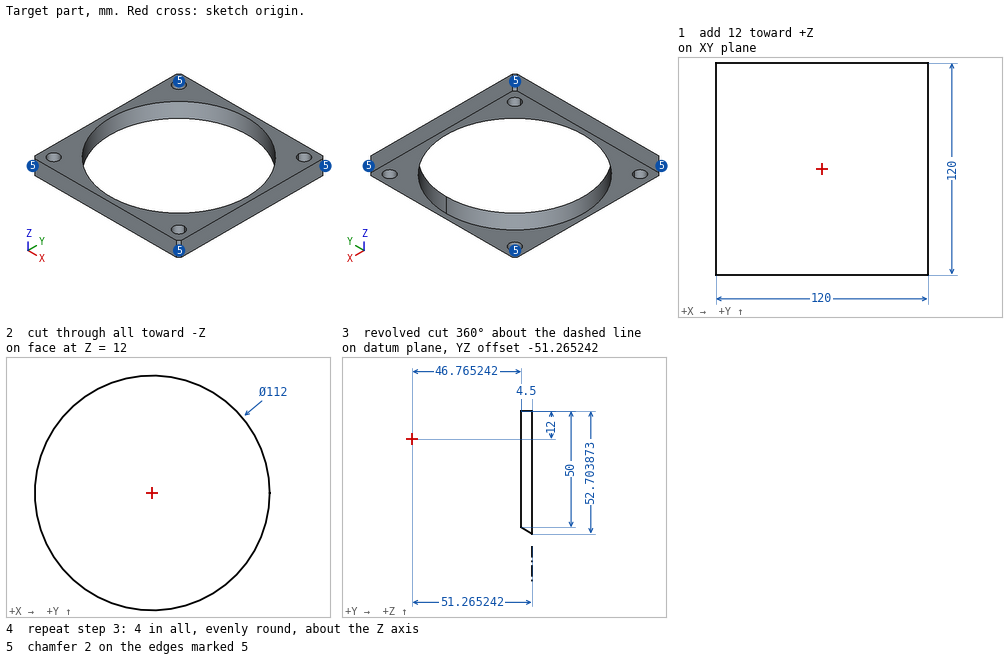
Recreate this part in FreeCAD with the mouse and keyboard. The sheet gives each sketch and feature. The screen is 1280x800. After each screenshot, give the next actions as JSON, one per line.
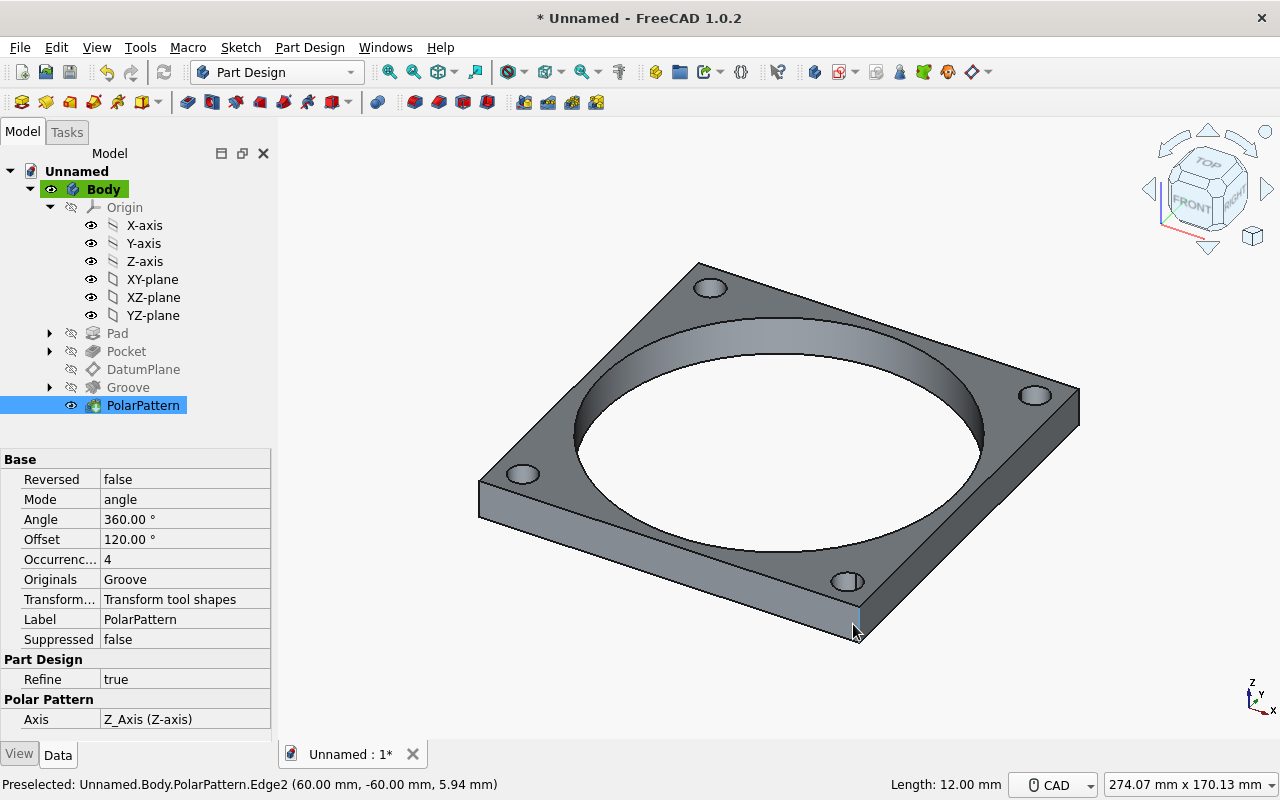
{"action": "key", "text": "0"}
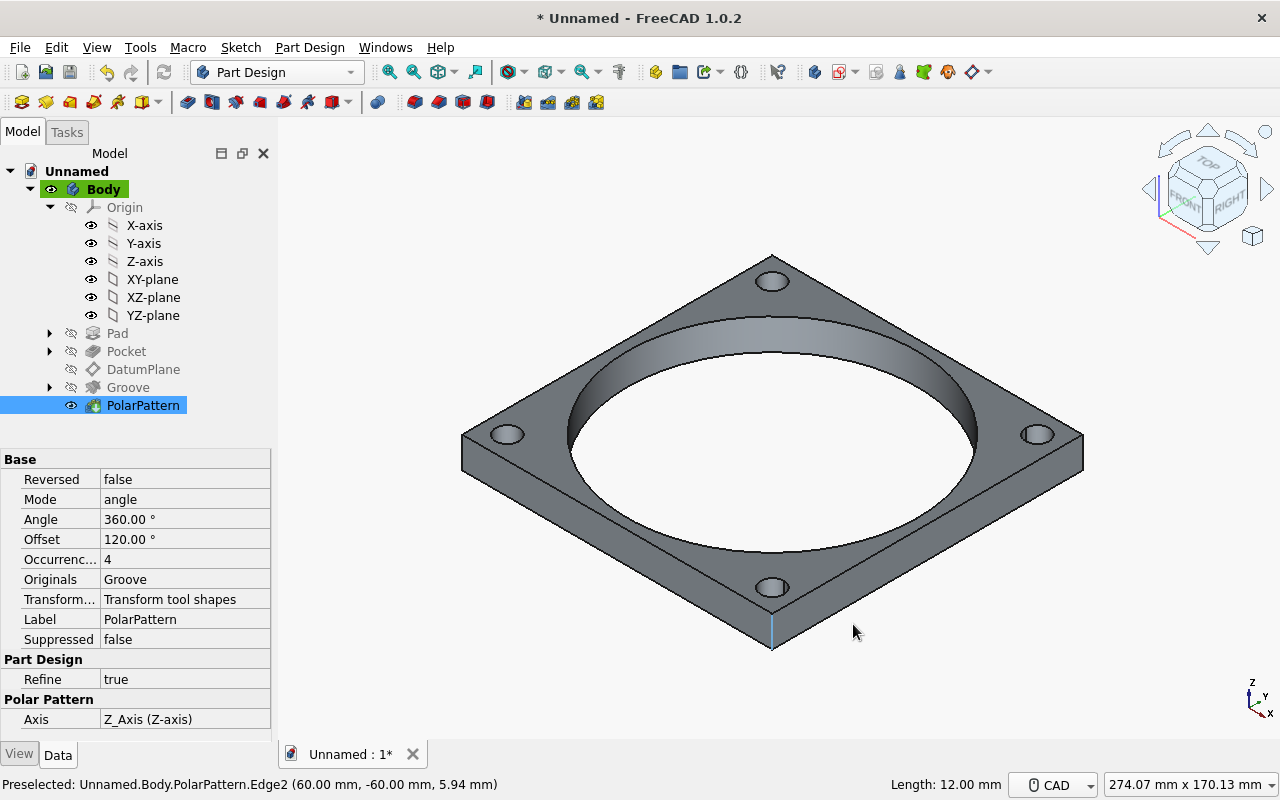
{"action": "key", "text": "2"}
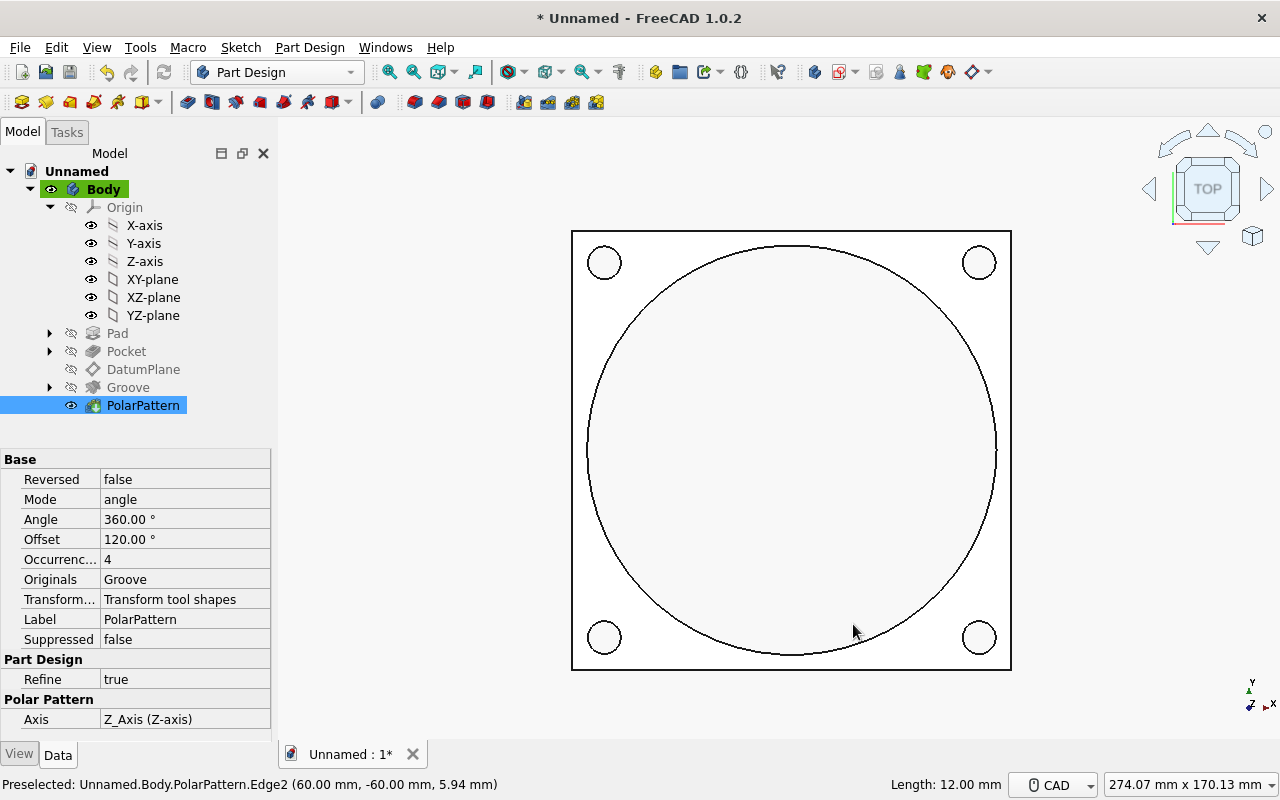
{"action": "key", "text": "1"}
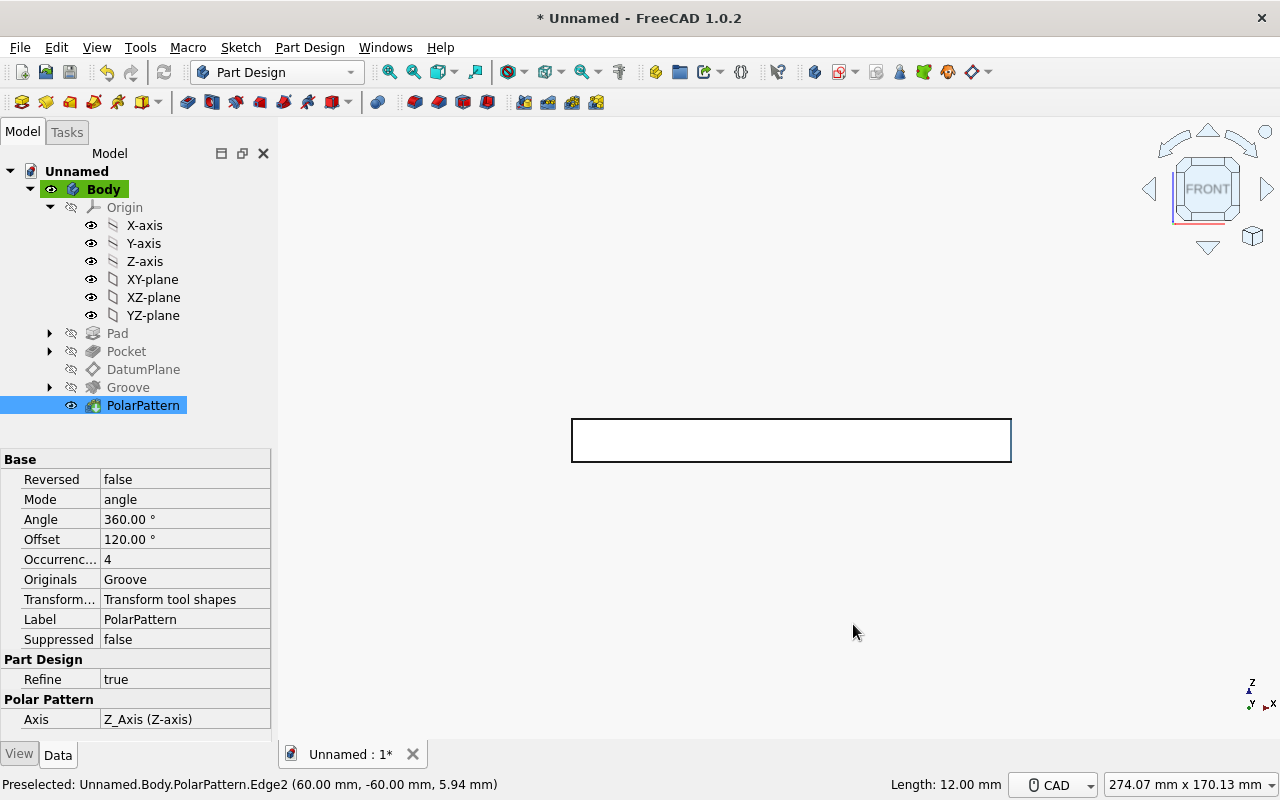
{"action": "left_click", "coordinate": [390, 72]}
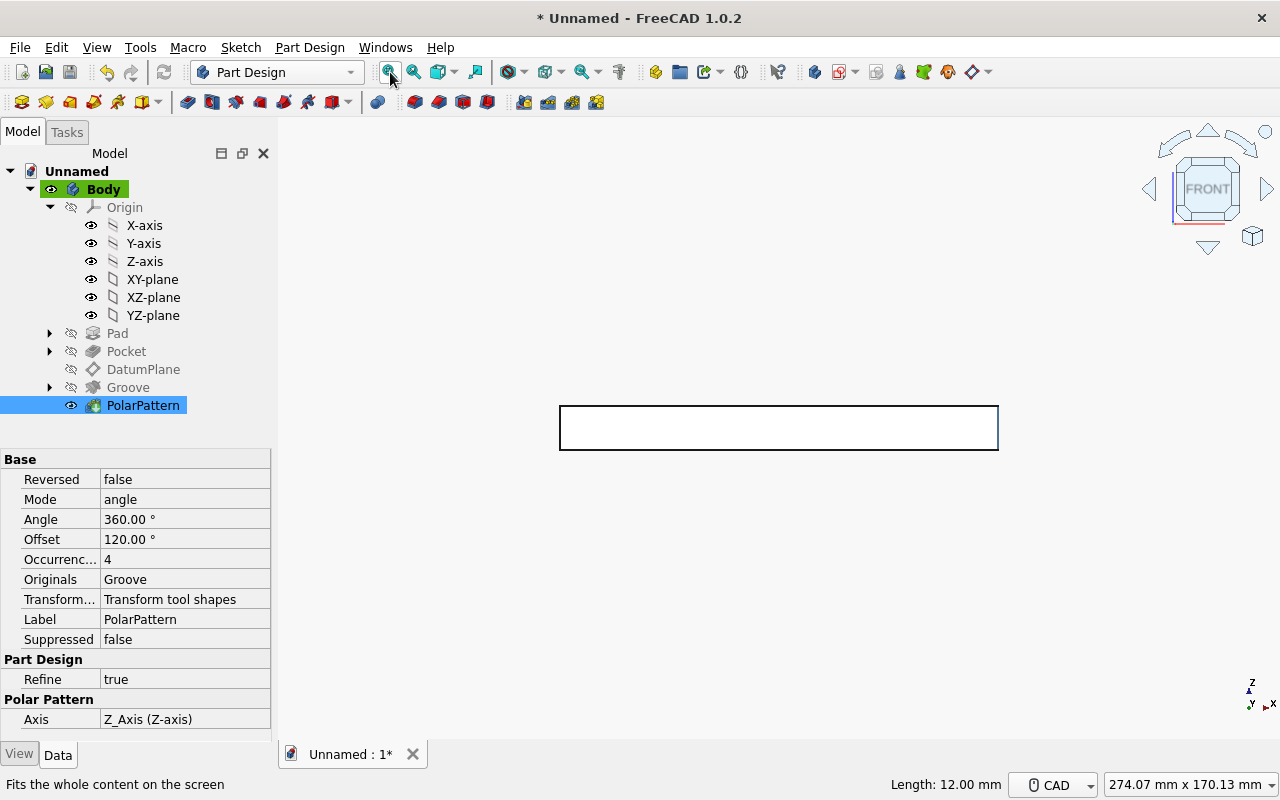
{"action": "left_click", "coordinate": [560, 427], "text": "ctrl"}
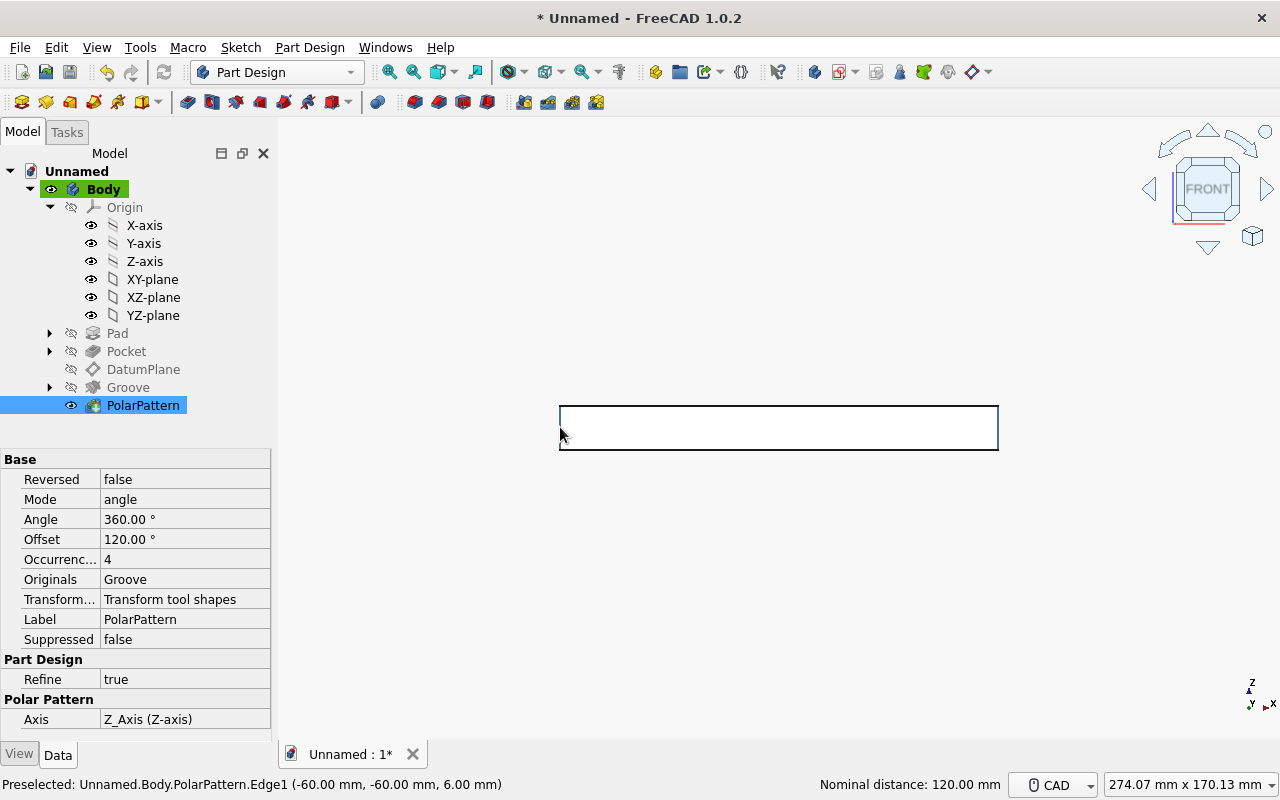
{"action": "key", "text": "3"}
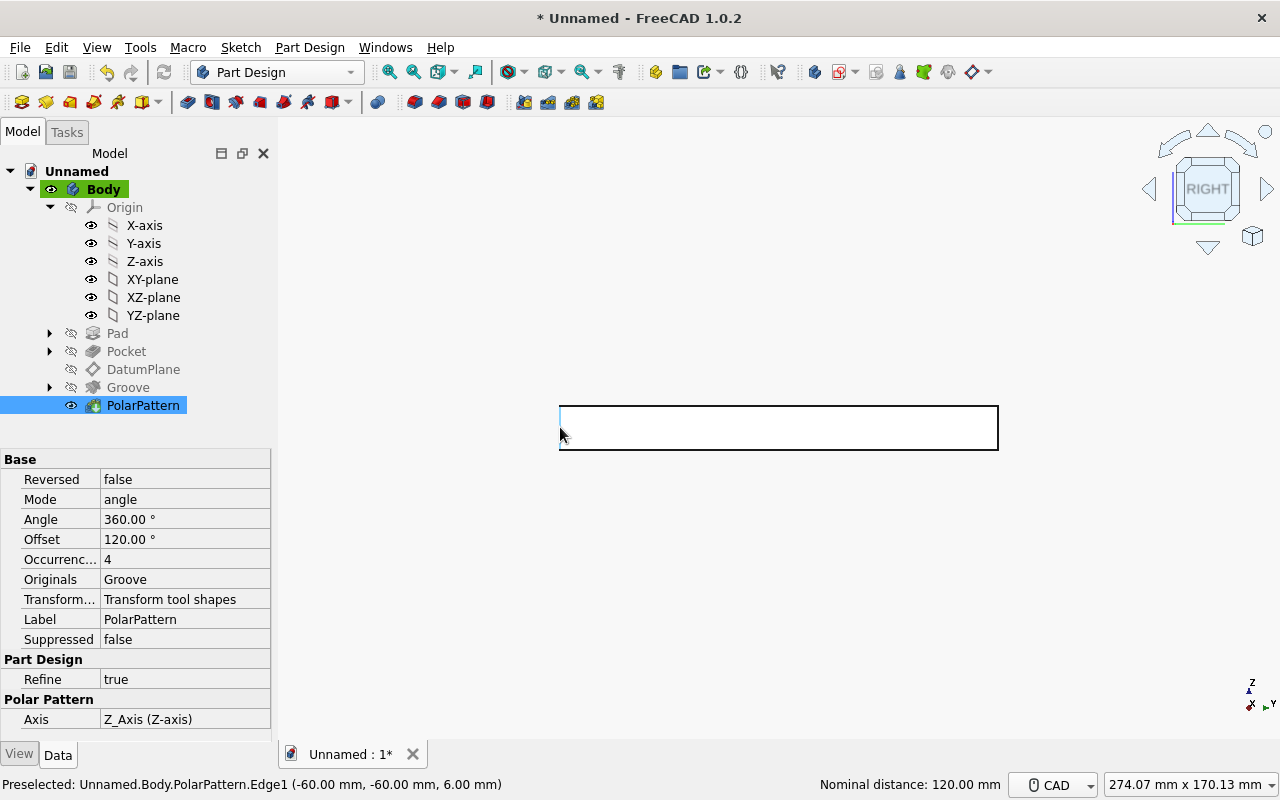
{"action": "key", "text": "v f"}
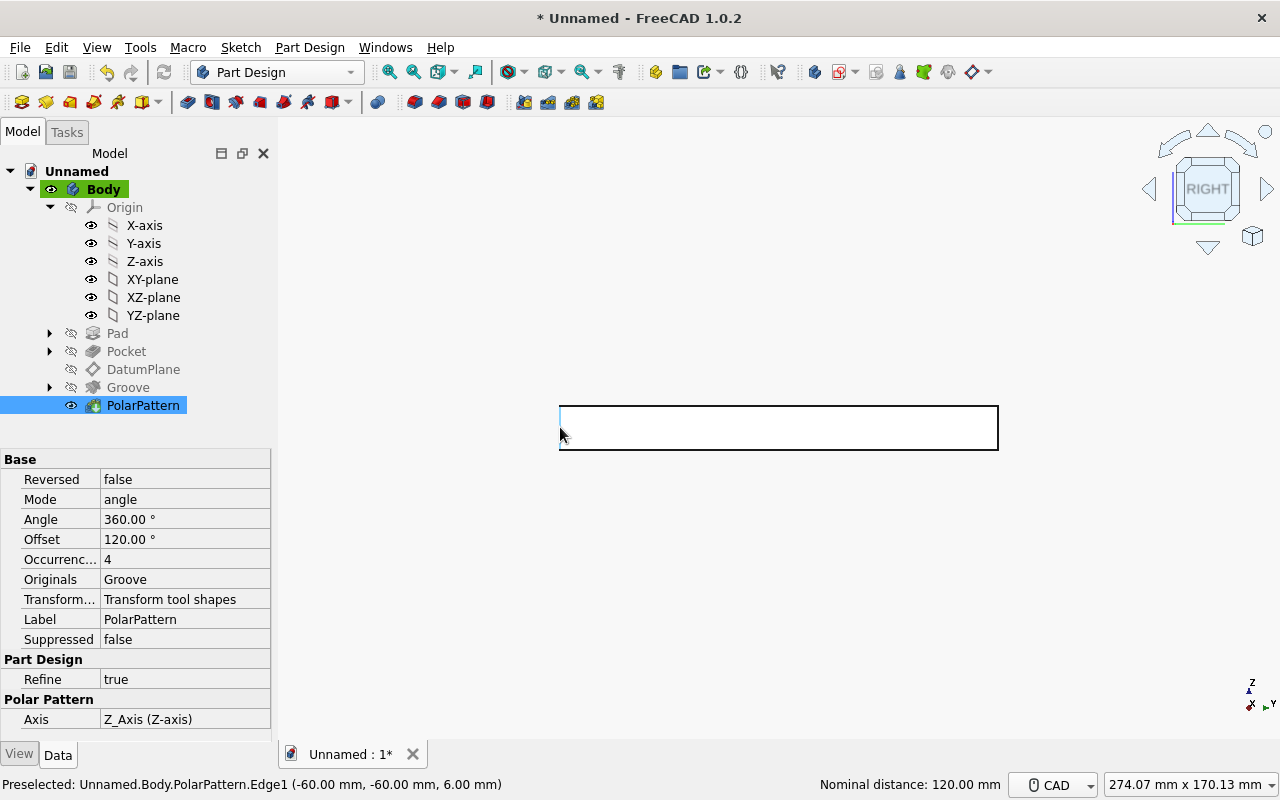
{"action": "left_click", "coordinate": [998, 427], "text": "ctrl"}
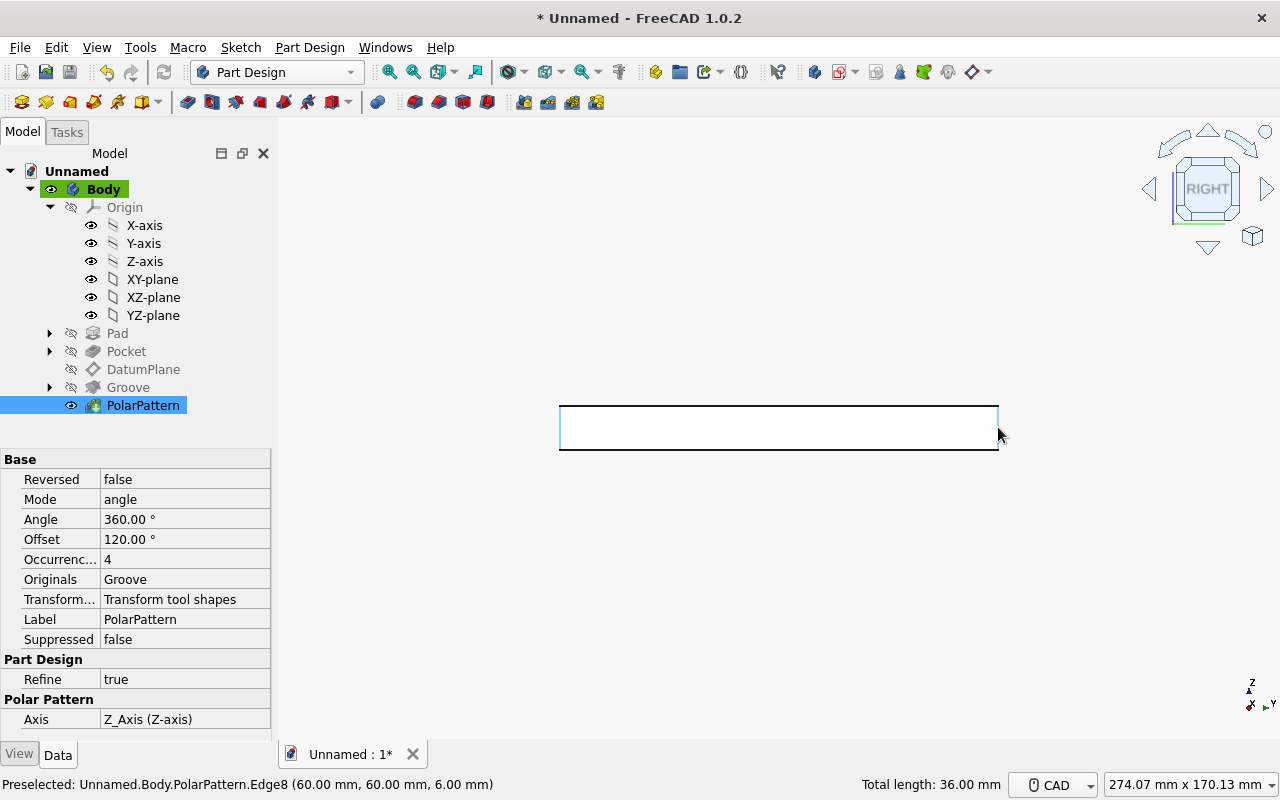
{"action": "key", "text": "5"}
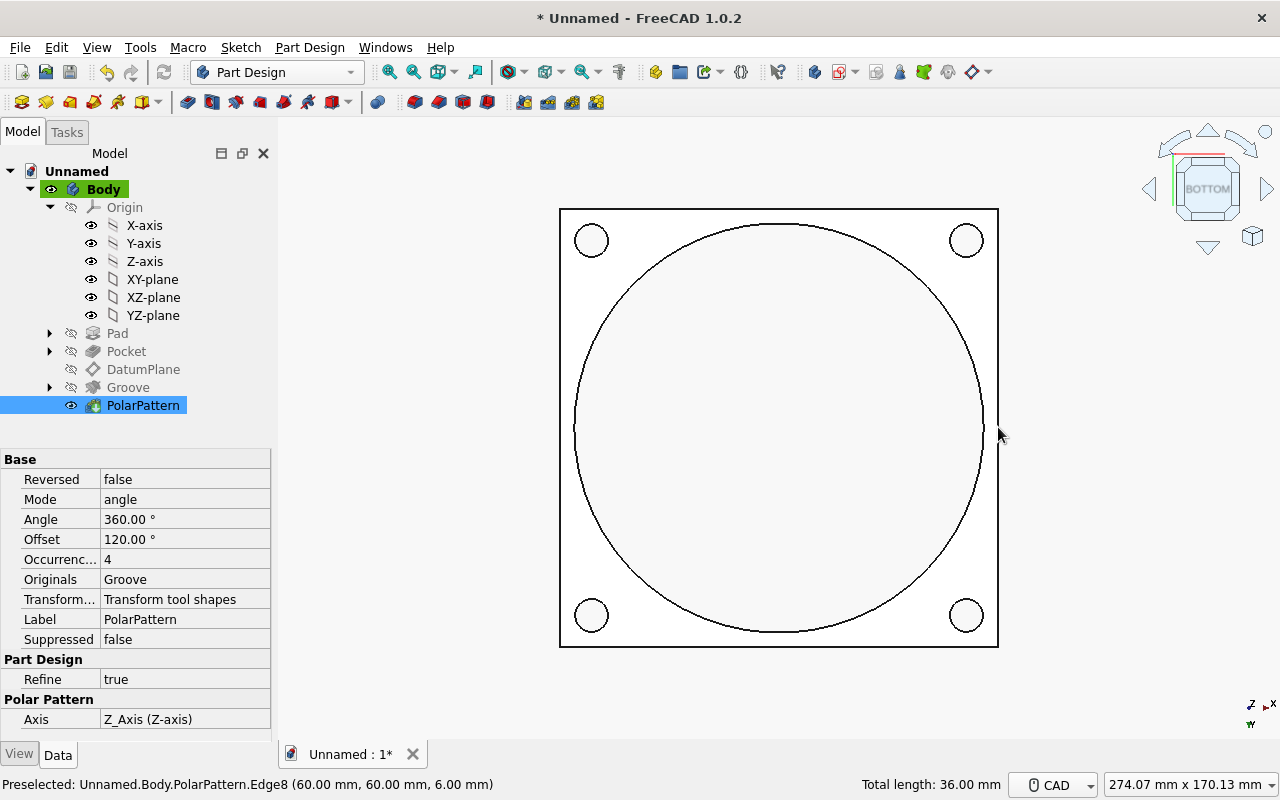
{"action": "key", "text": "4"}